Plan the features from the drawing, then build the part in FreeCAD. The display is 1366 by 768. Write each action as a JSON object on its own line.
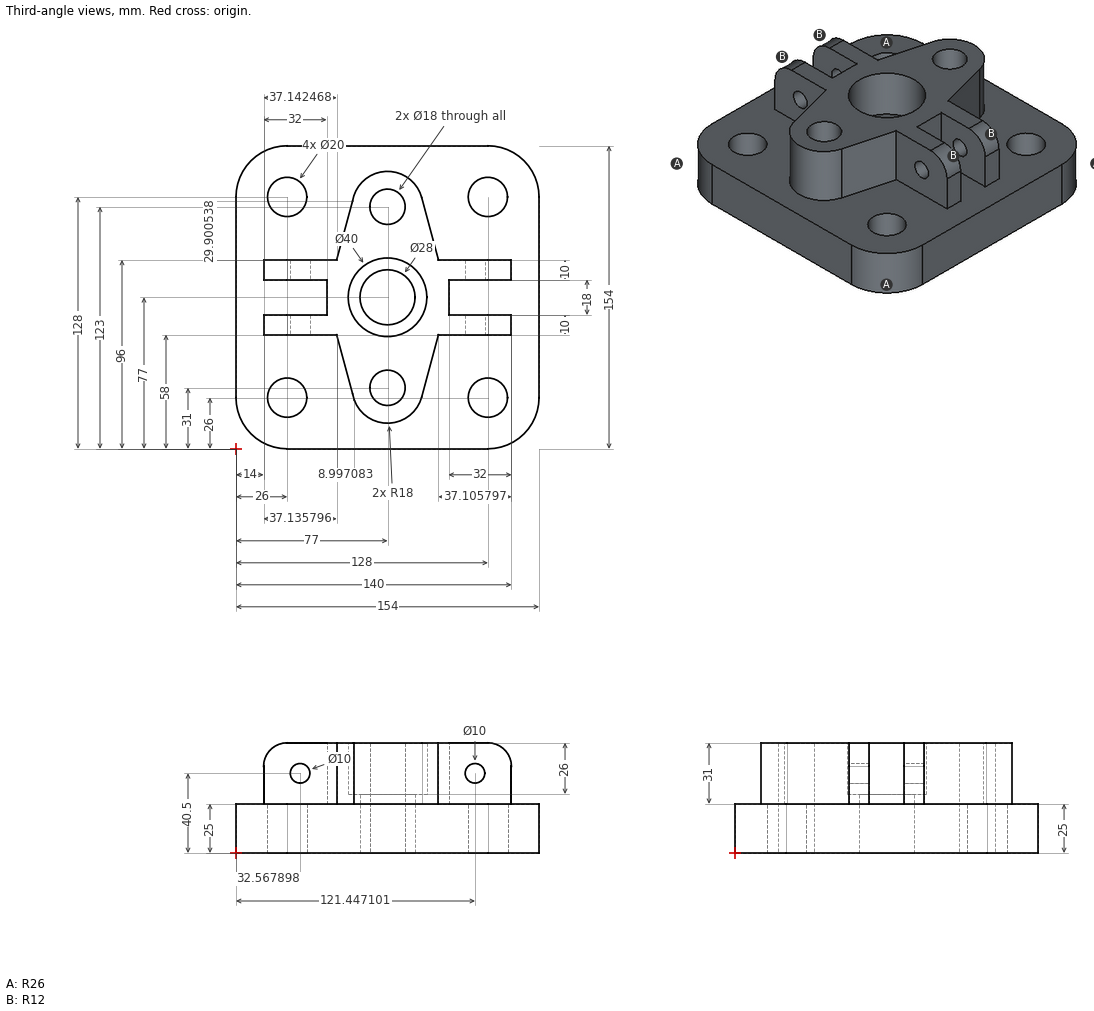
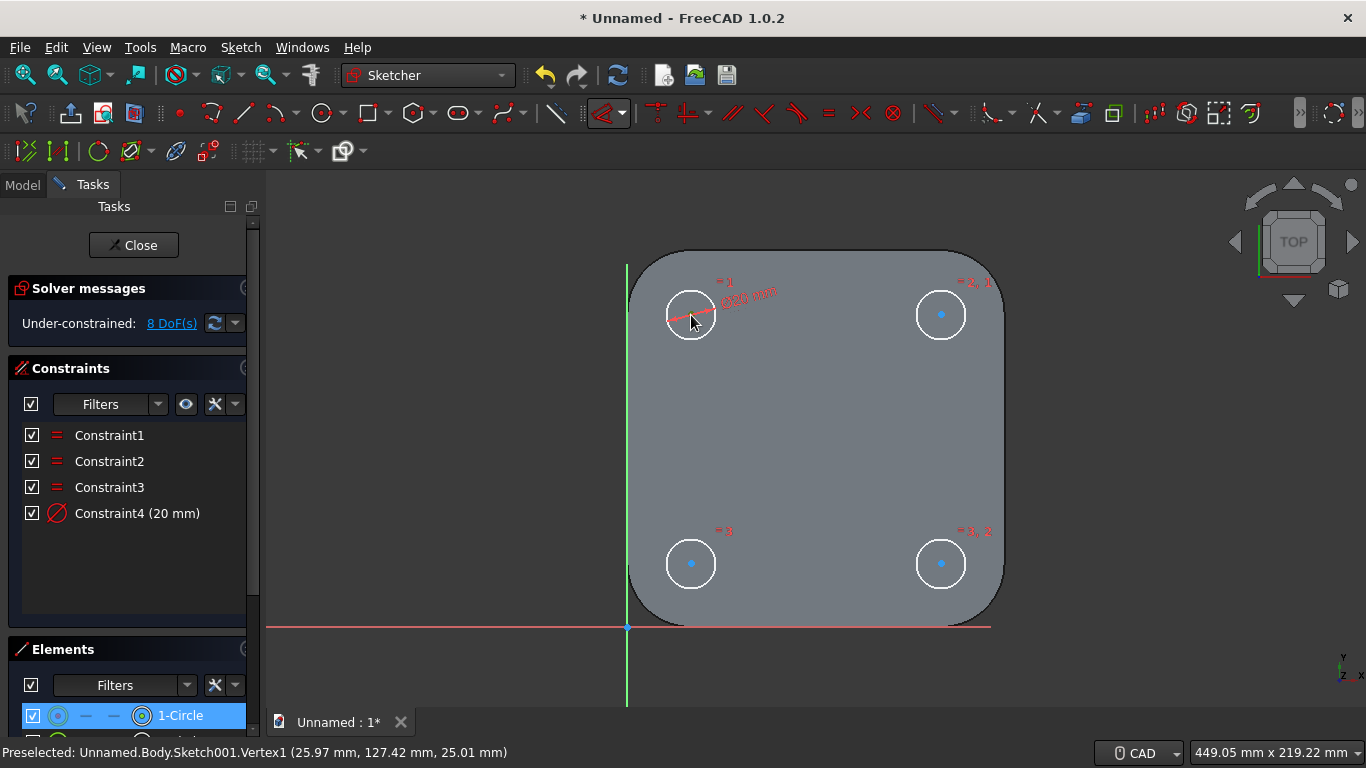
{"action": "key", "text": "l"}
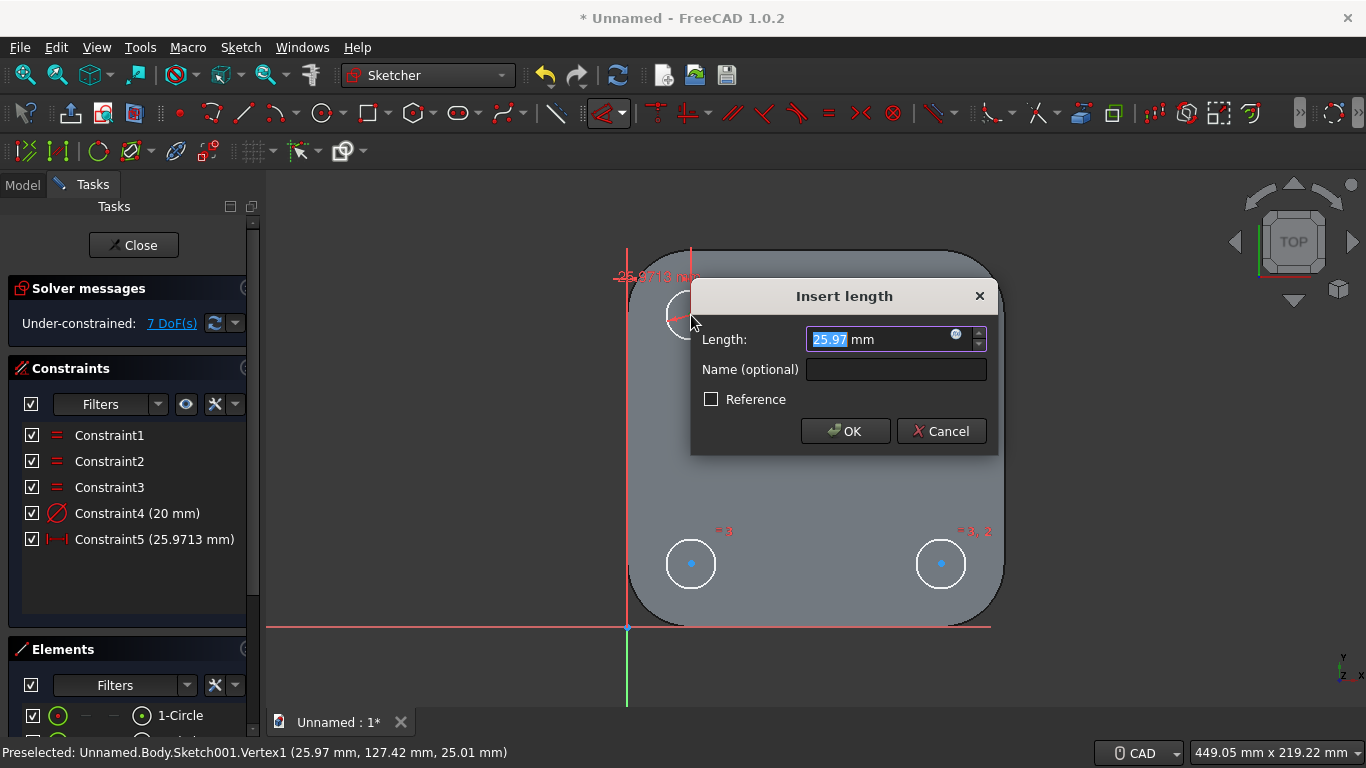
{"action": "type", "text": "26"}
{"action": "key", "text": "Return"}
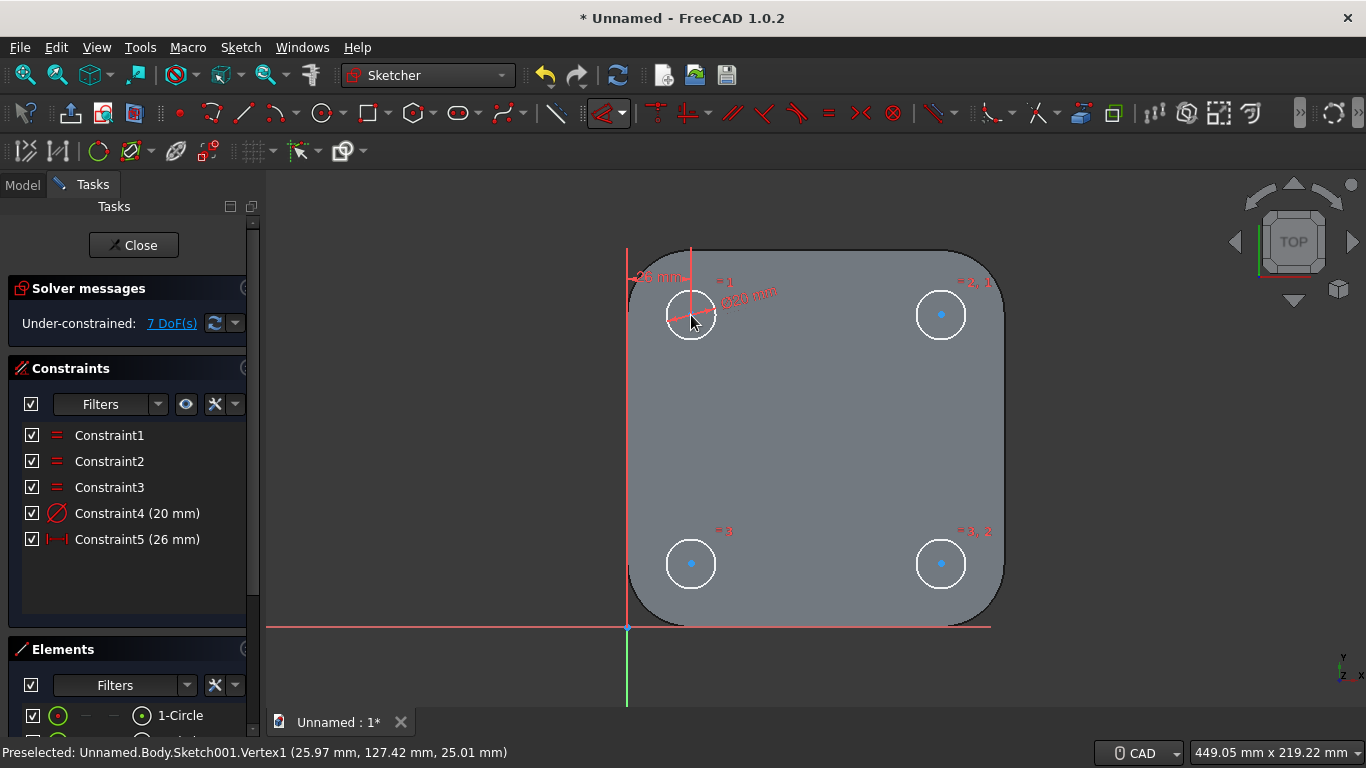
{"action": "left_click", "coordinate": [941, 564]}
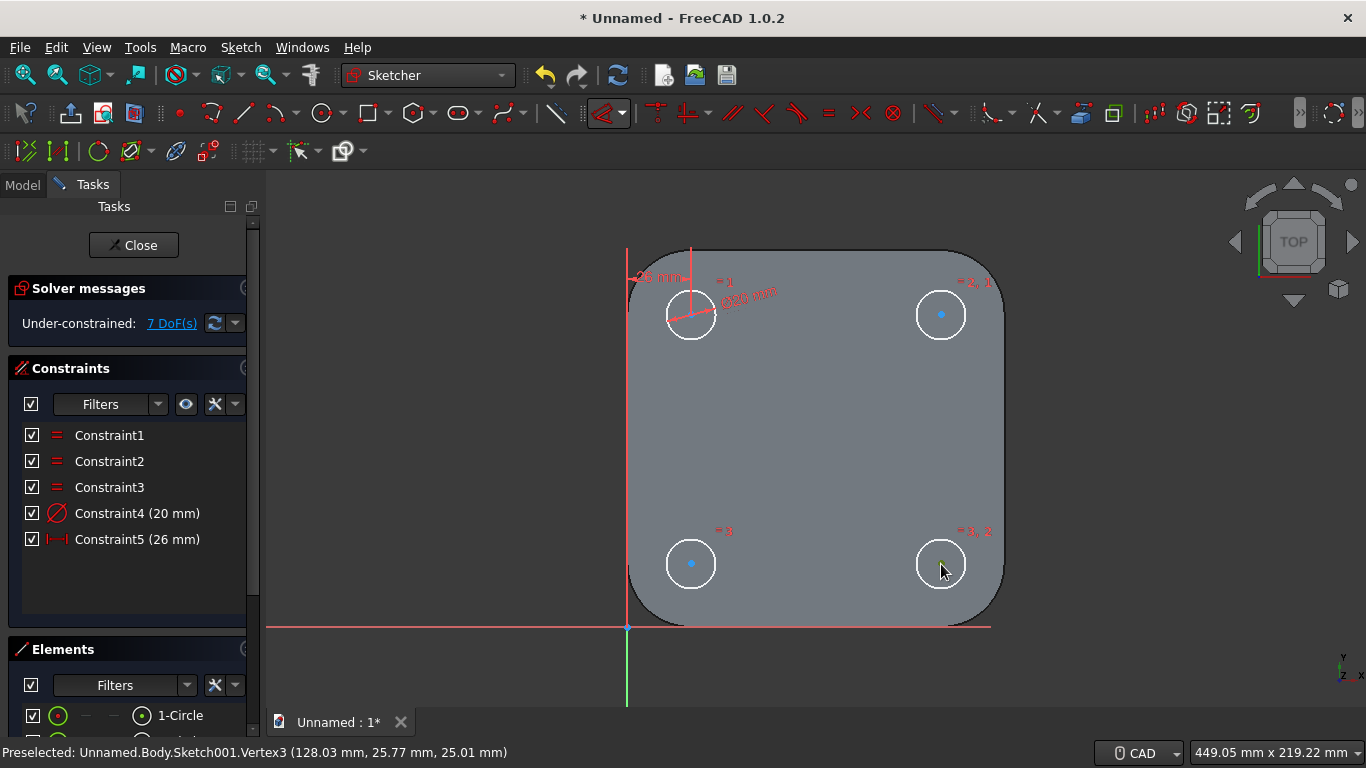
{"action": "key", "text": "i"}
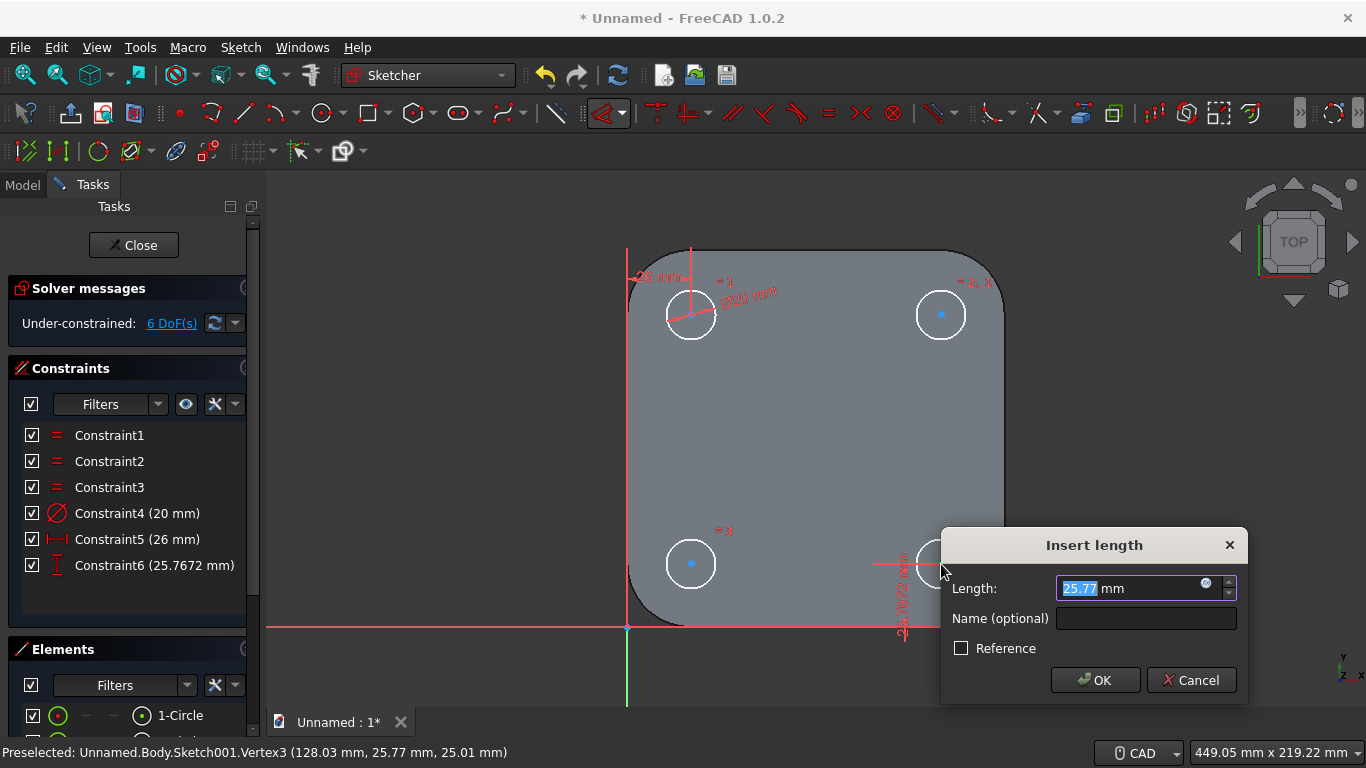
{"action": "type", "text": "26"}
{"action": "key", "text": "Return"}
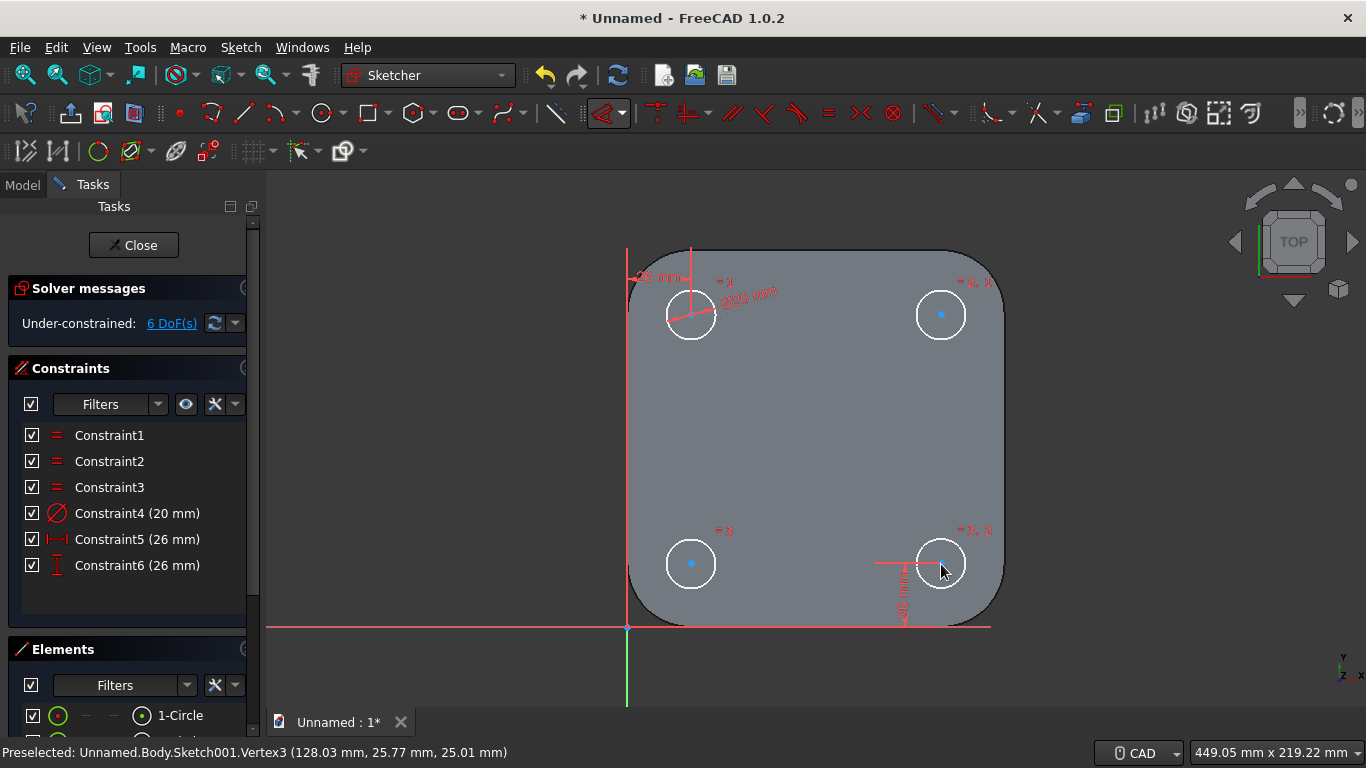
{"action": "left_click", "coordinate": [691, 564]}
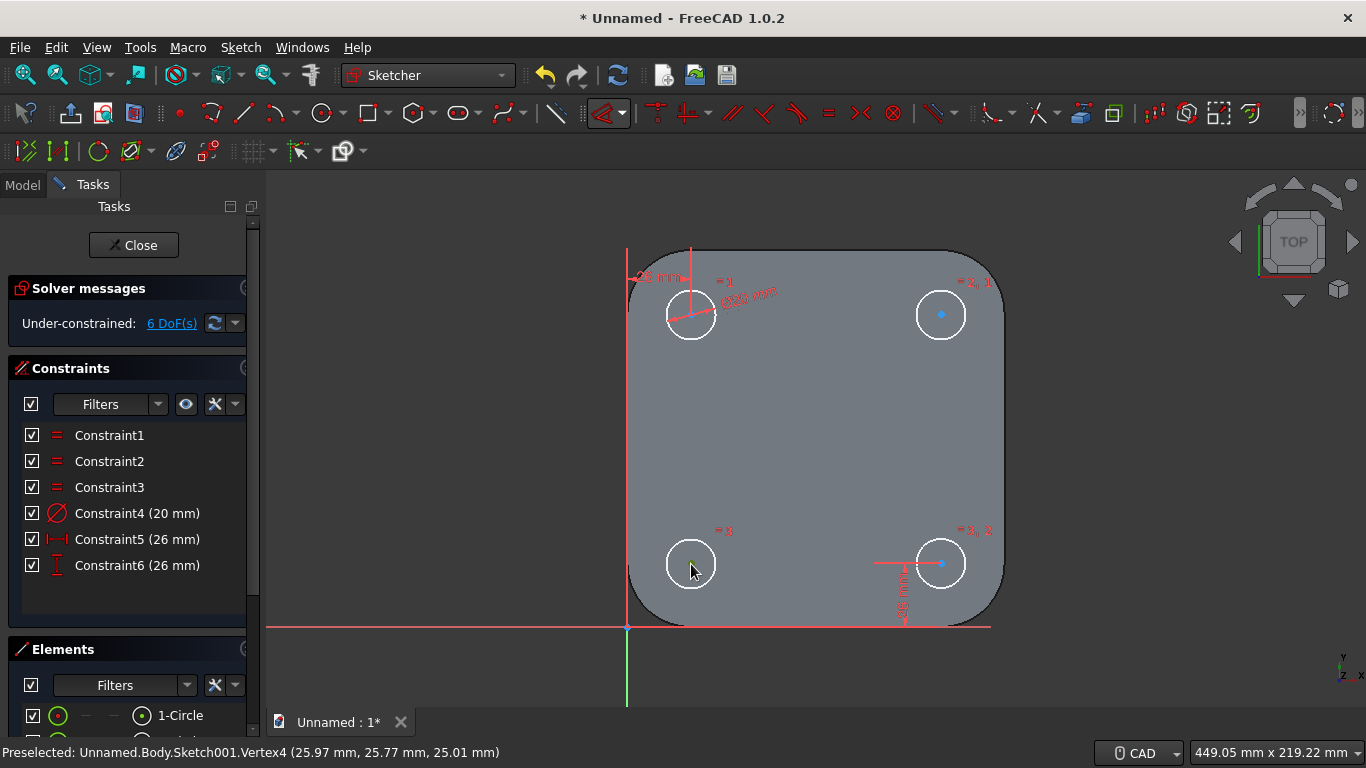
{"action": "key", "text": "l"}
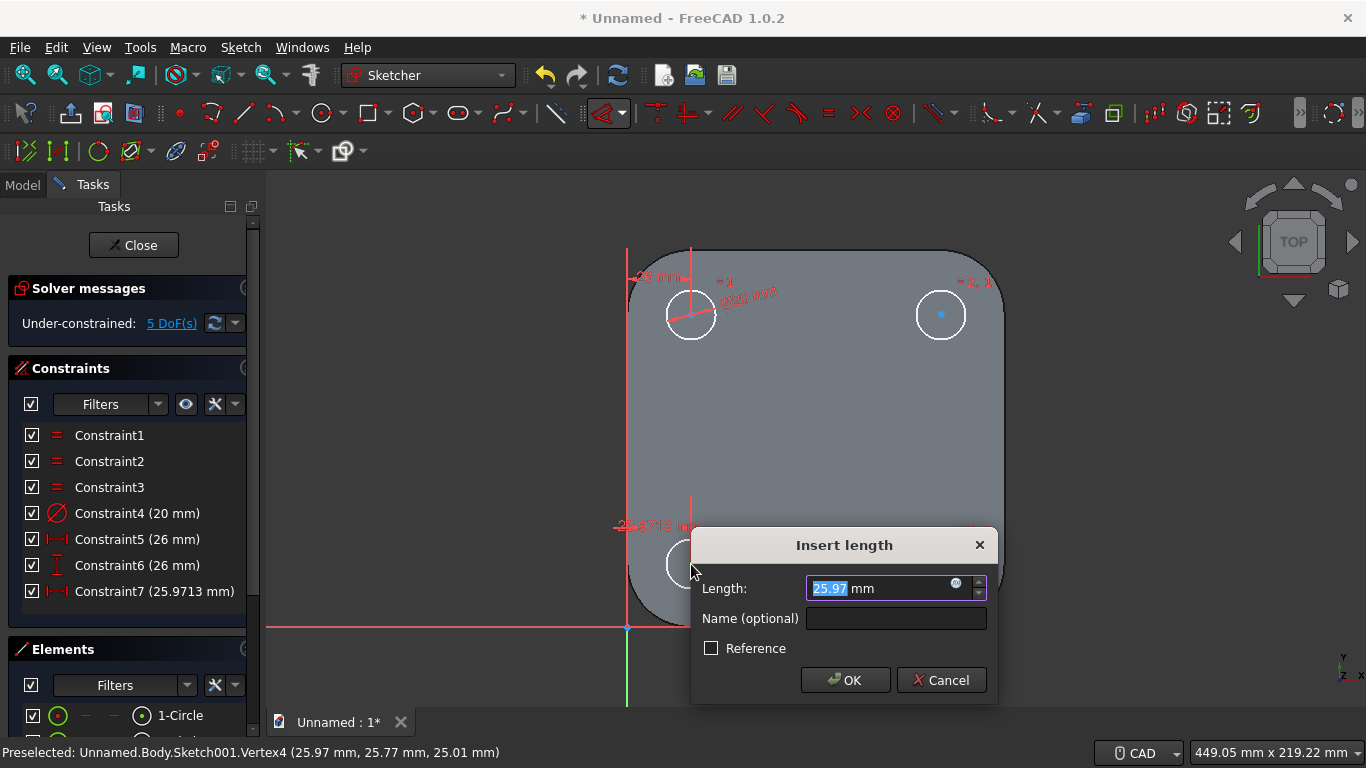
{"action": "type", "text": "26"}
{"action": "key", "text": "Return"}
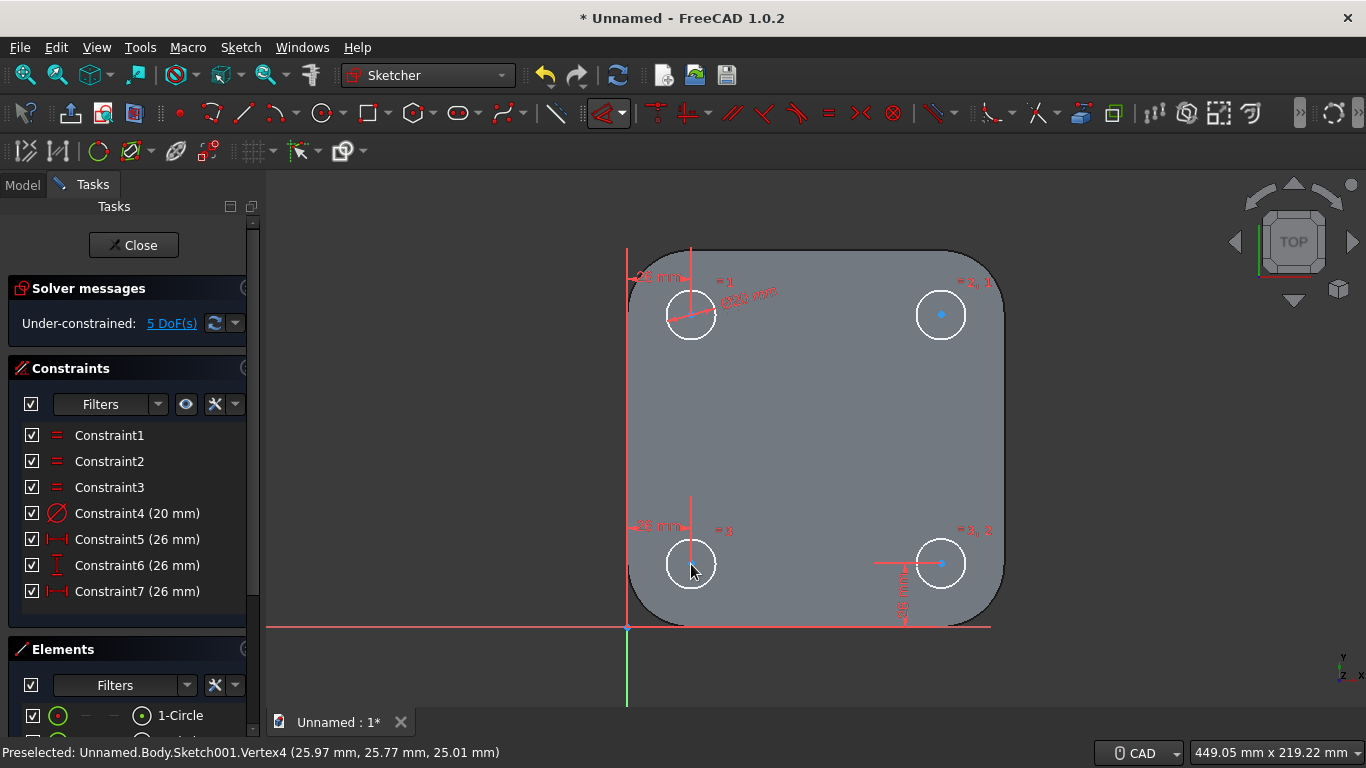
{"action": "left_click", "coordinate": [691, 564]}